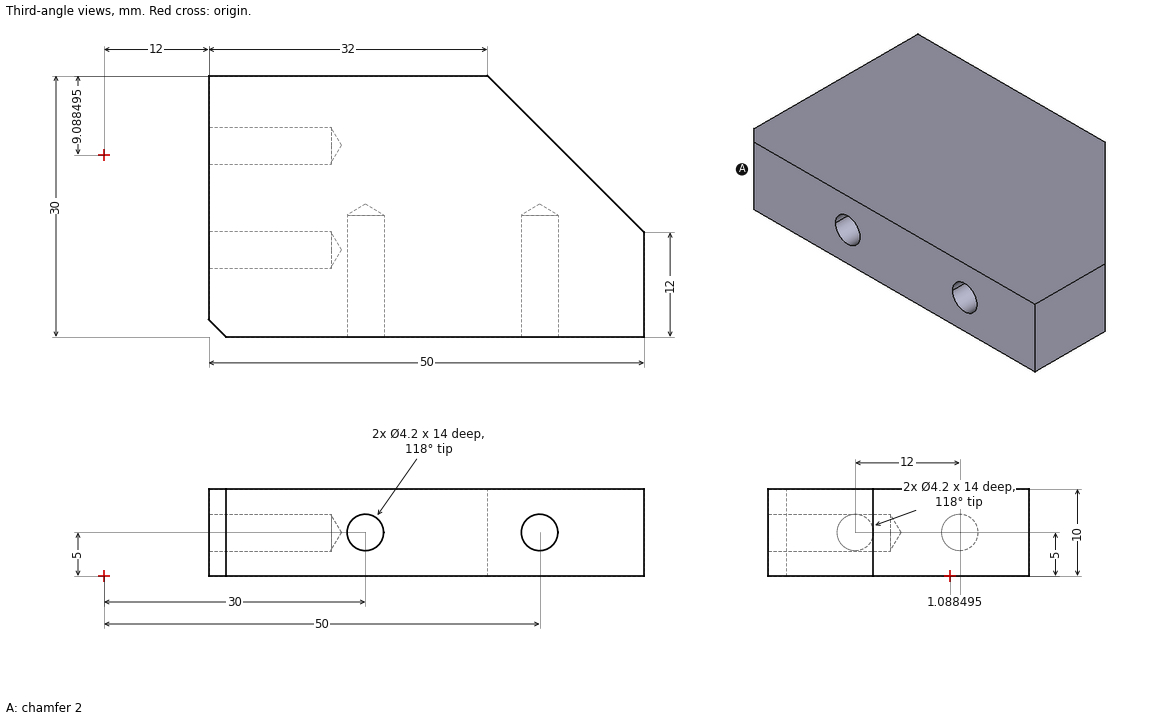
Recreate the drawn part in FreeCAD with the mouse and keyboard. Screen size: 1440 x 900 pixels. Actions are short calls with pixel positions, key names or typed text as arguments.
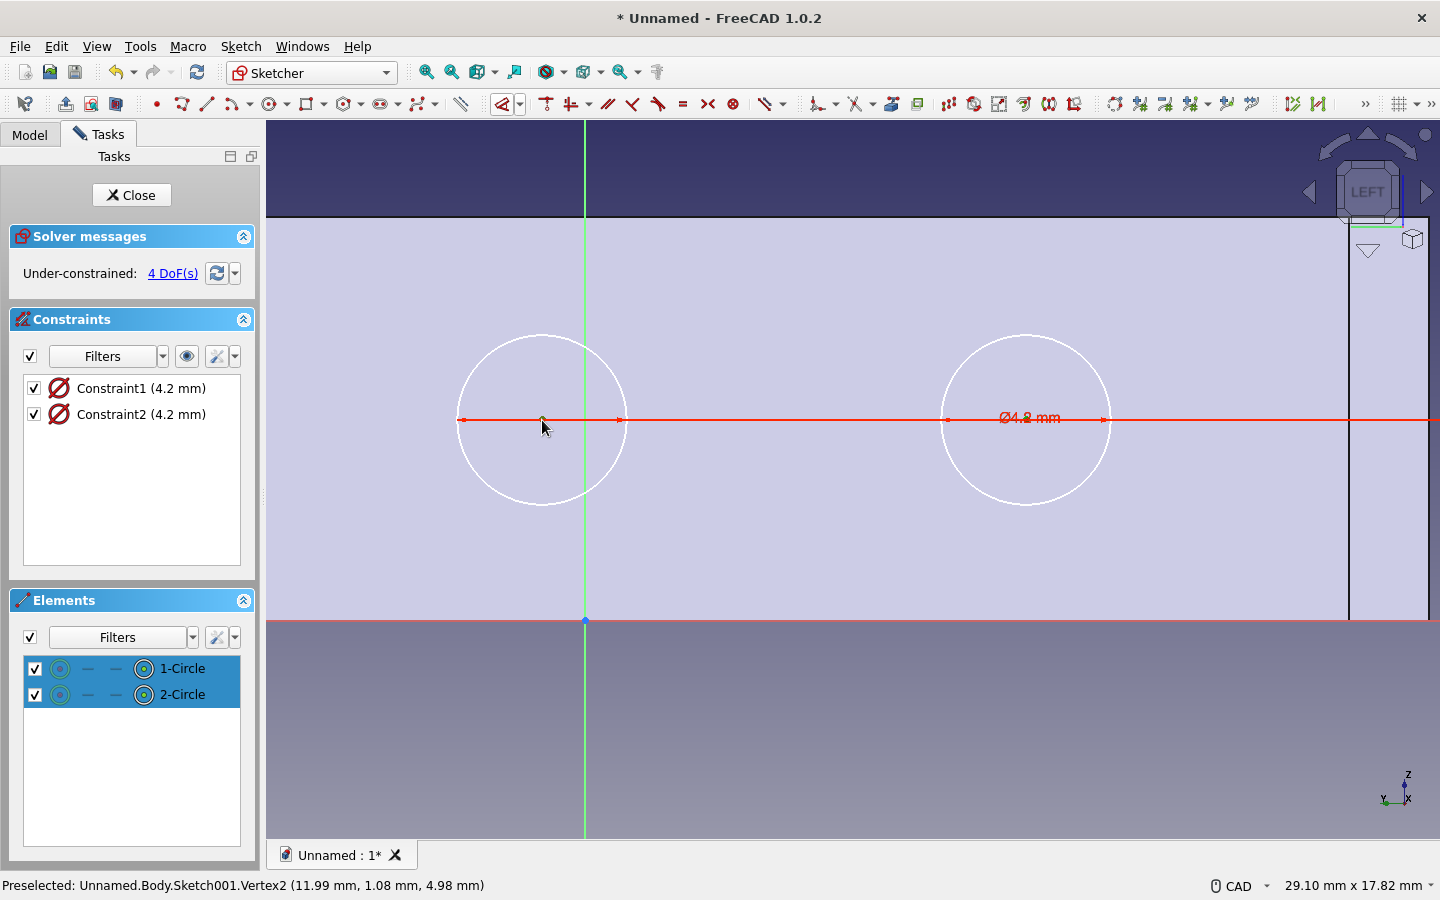
key(h)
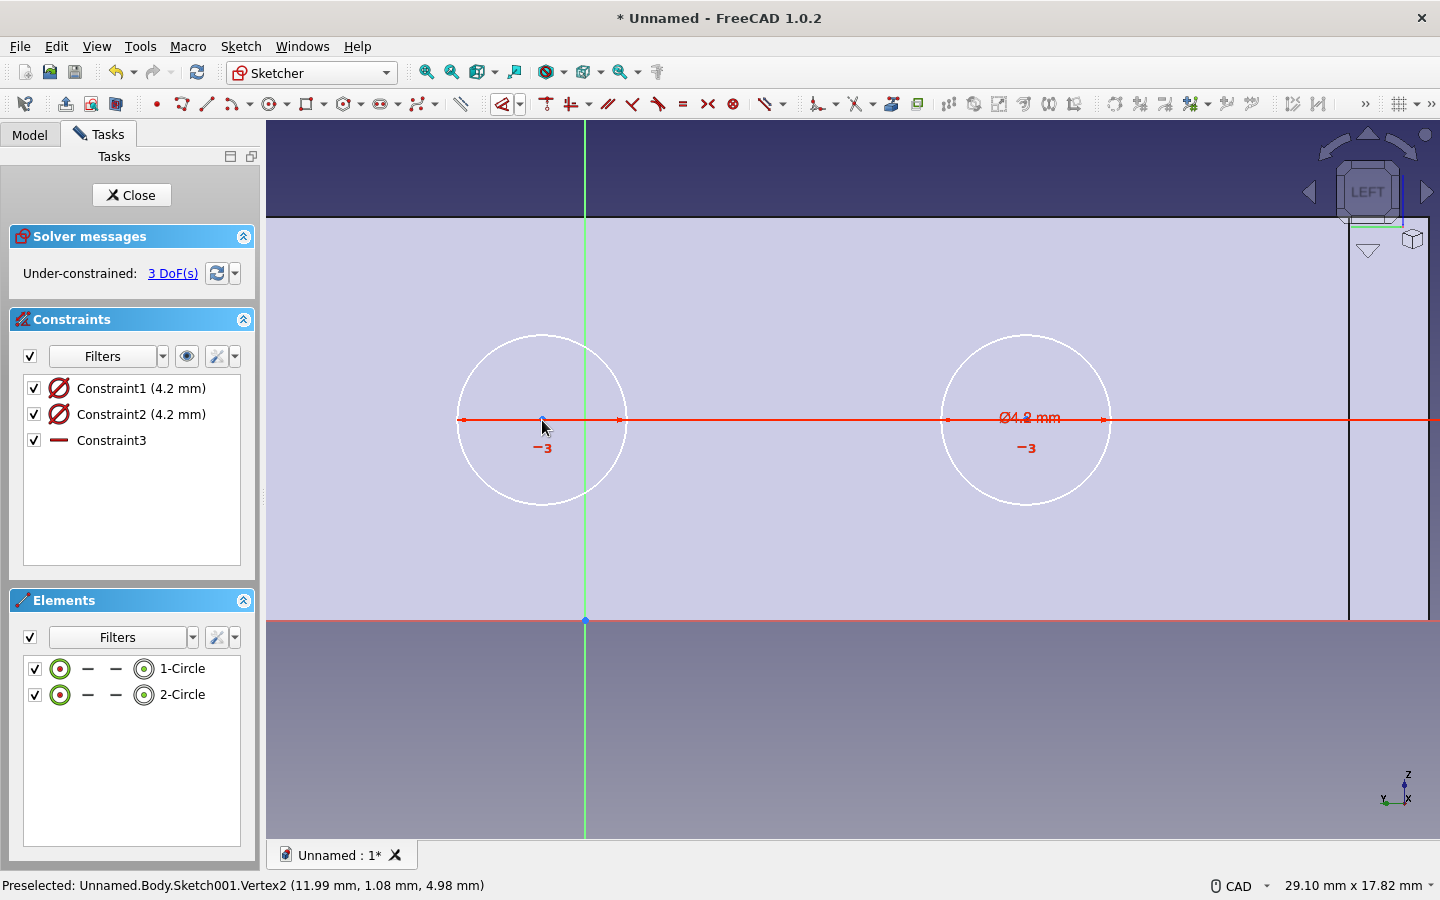
click(1026, 420)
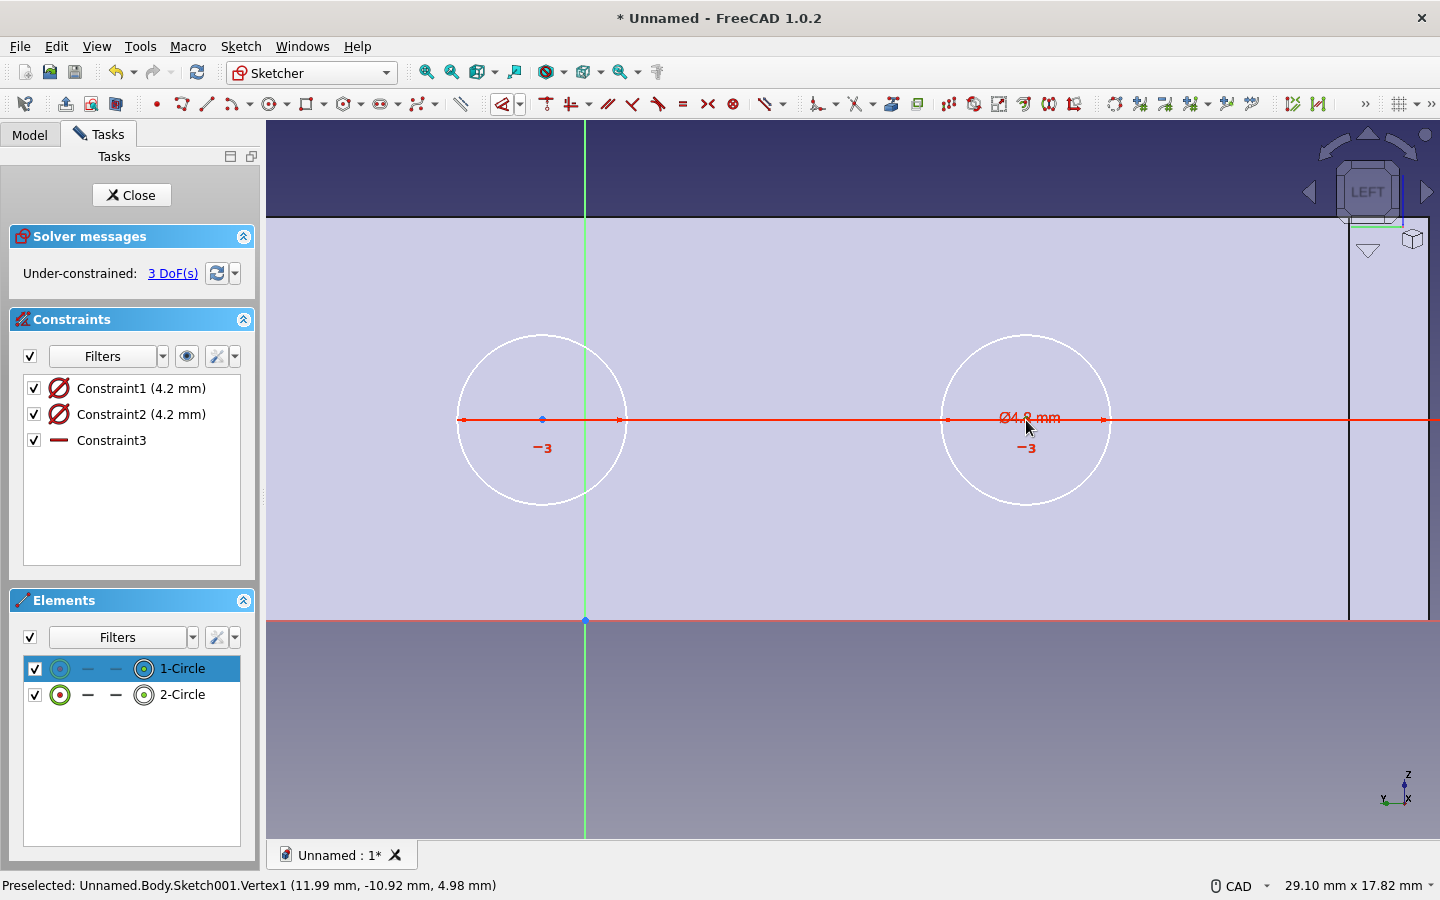
key(i)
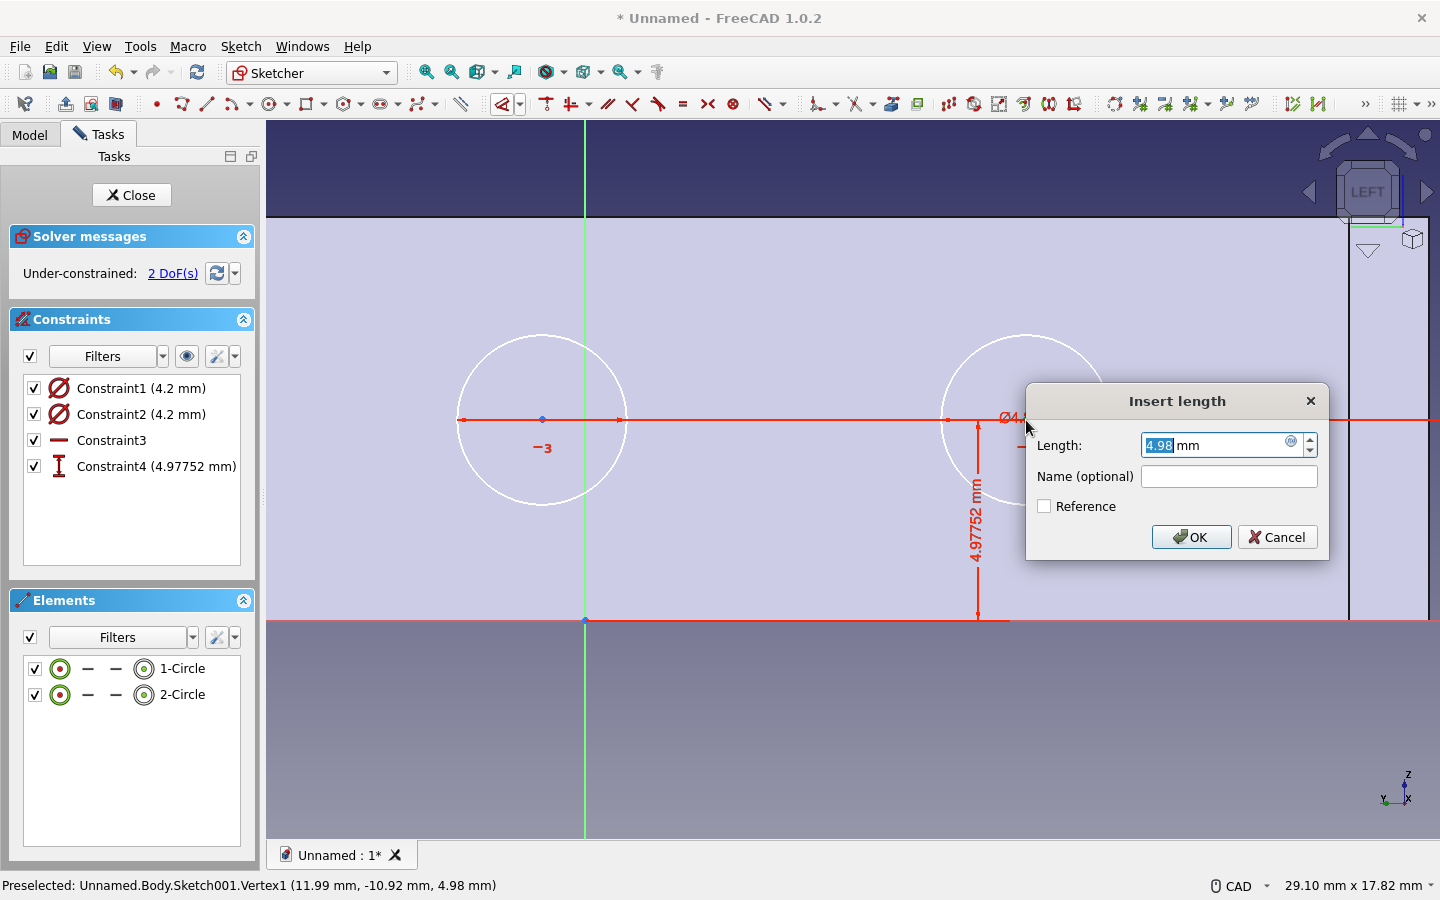
text(5)
key(Return)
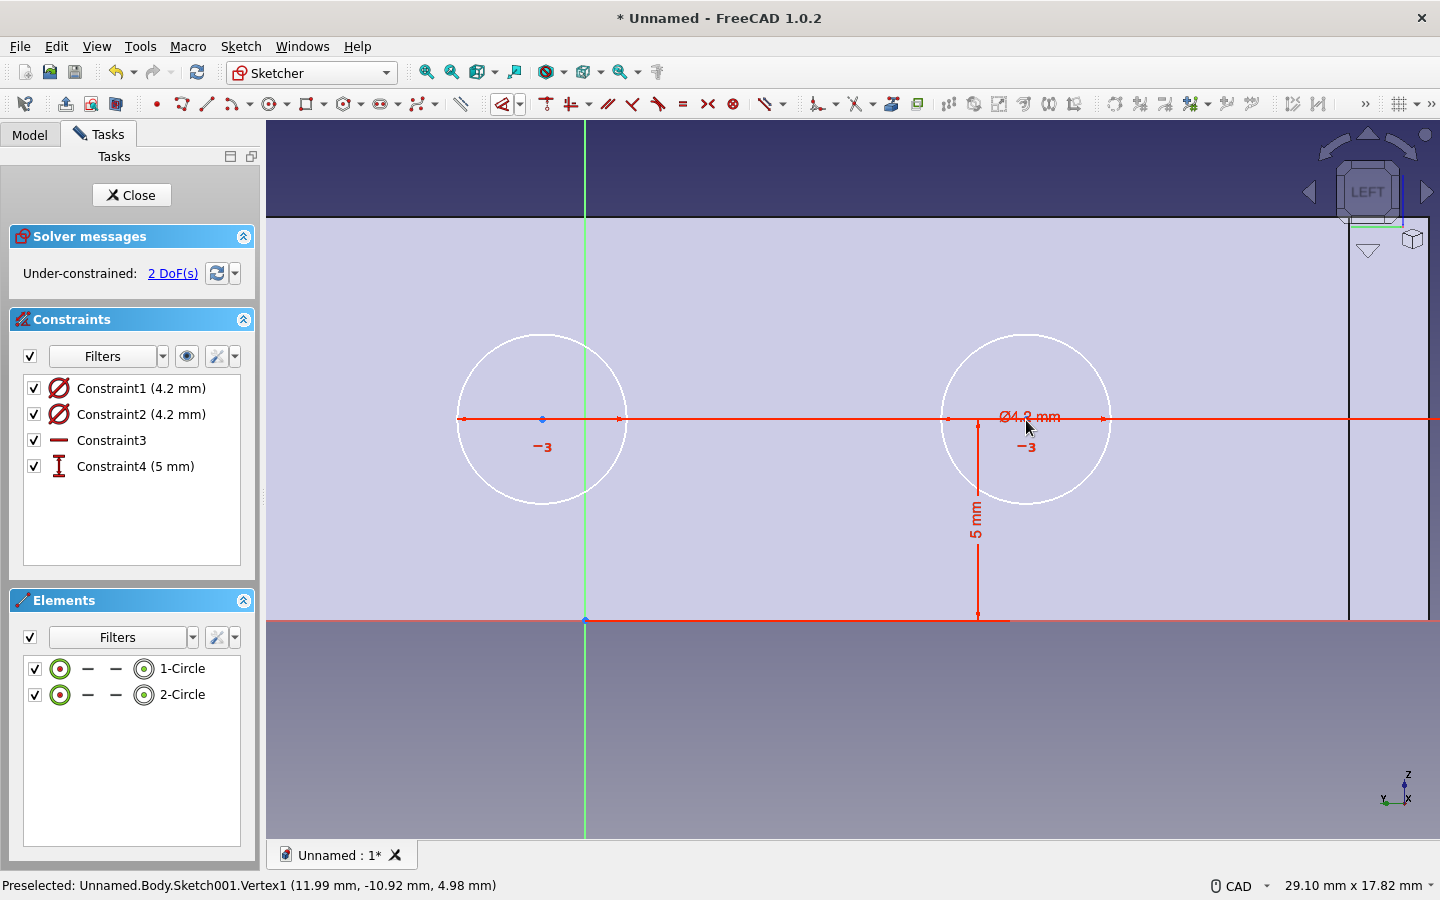
click(1026, 419)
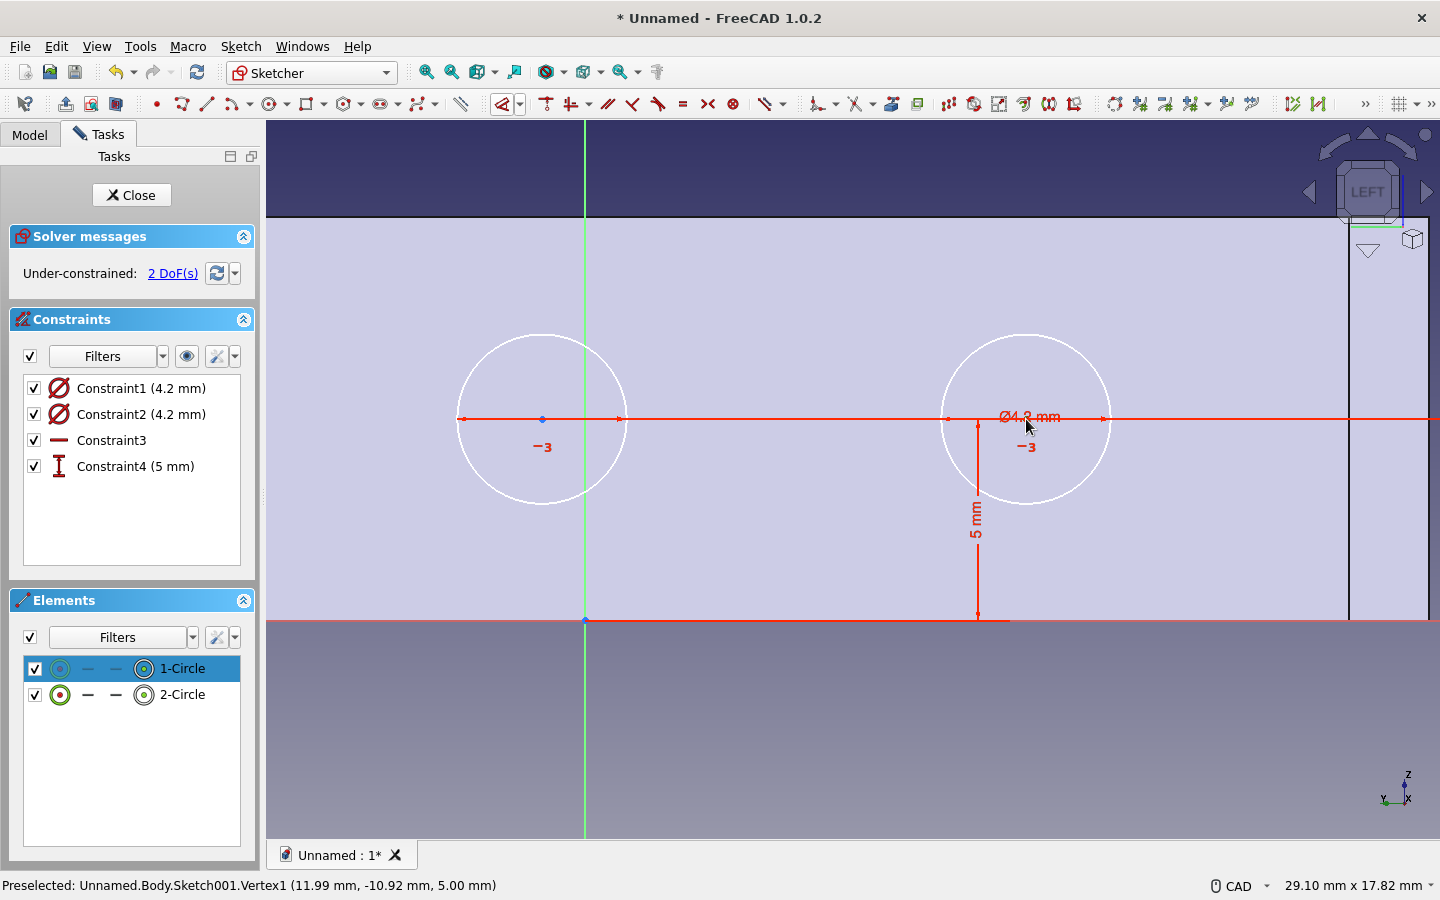
click(542, 419)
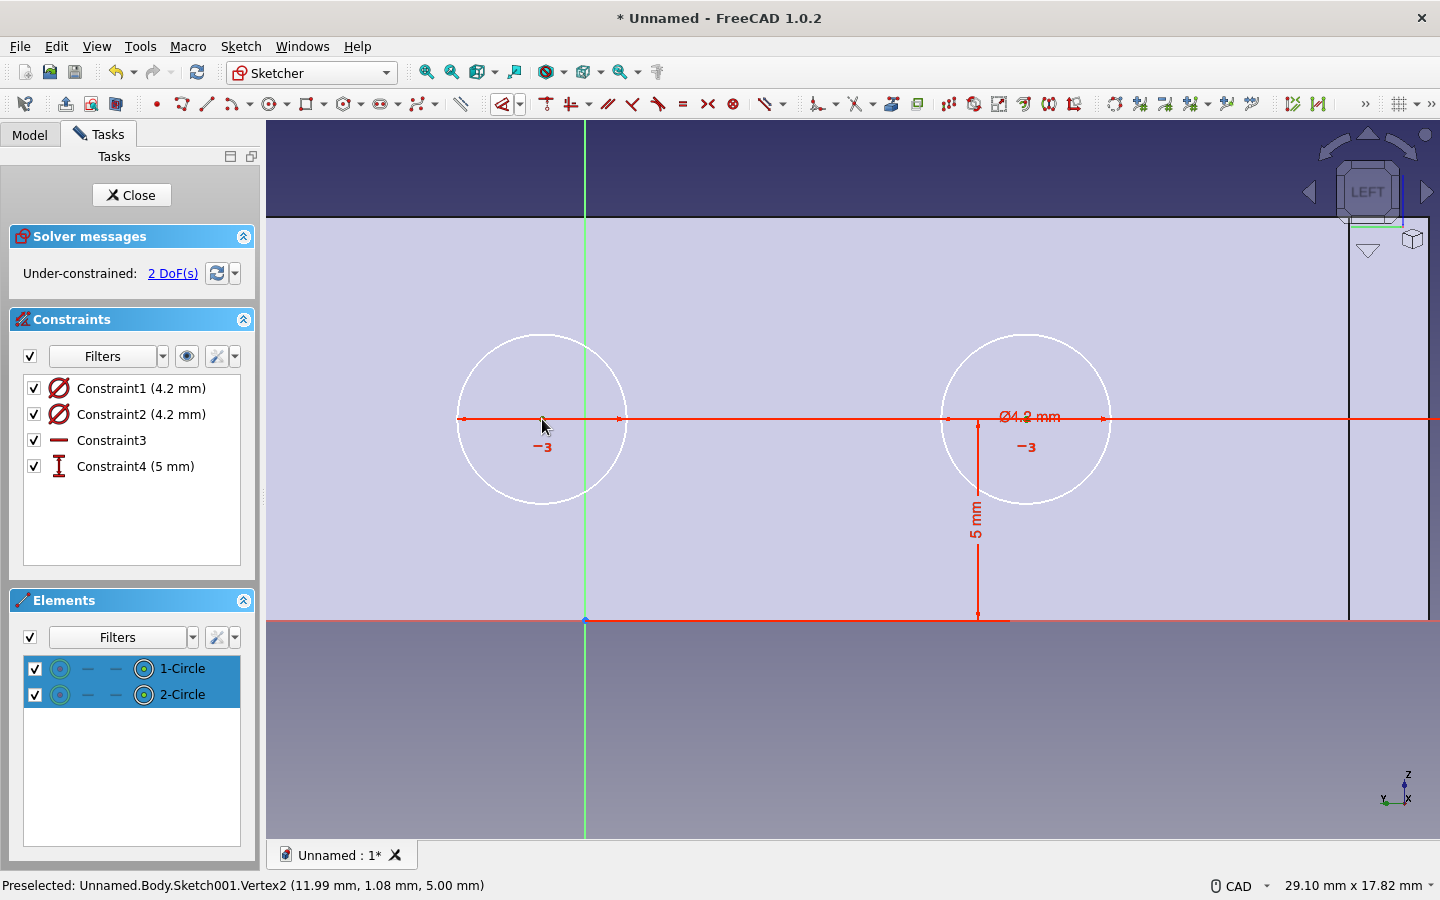
key(l)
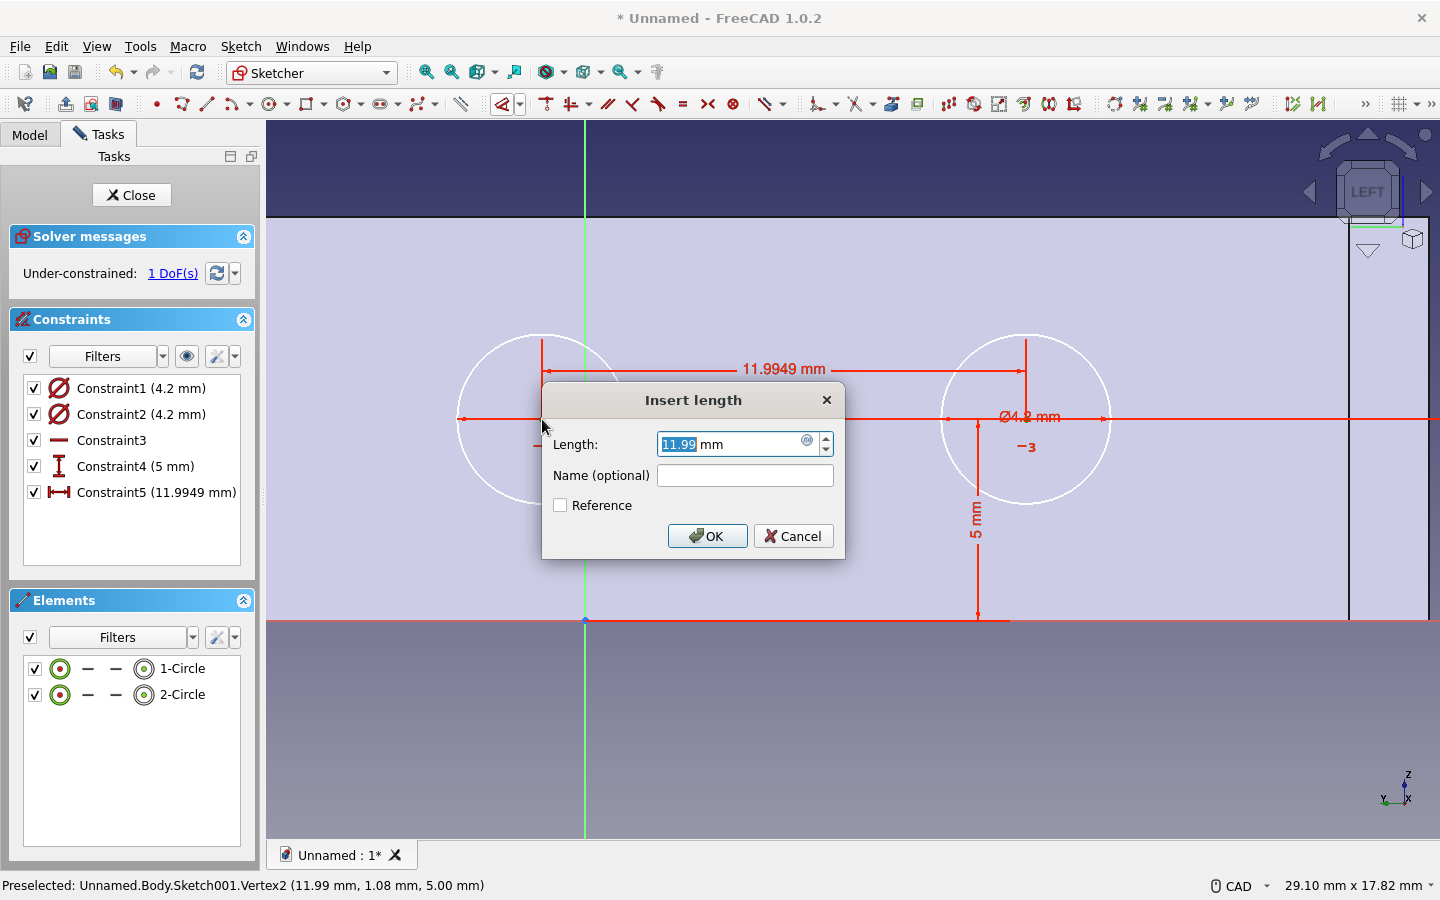
text(12)
key(Return)